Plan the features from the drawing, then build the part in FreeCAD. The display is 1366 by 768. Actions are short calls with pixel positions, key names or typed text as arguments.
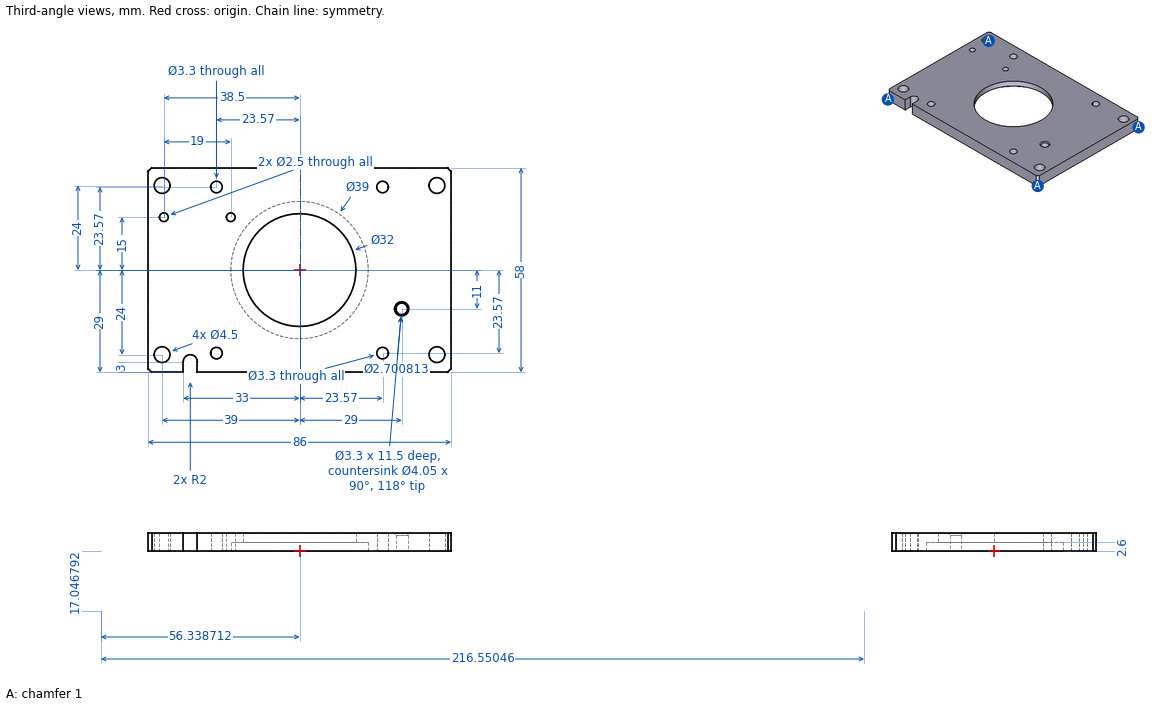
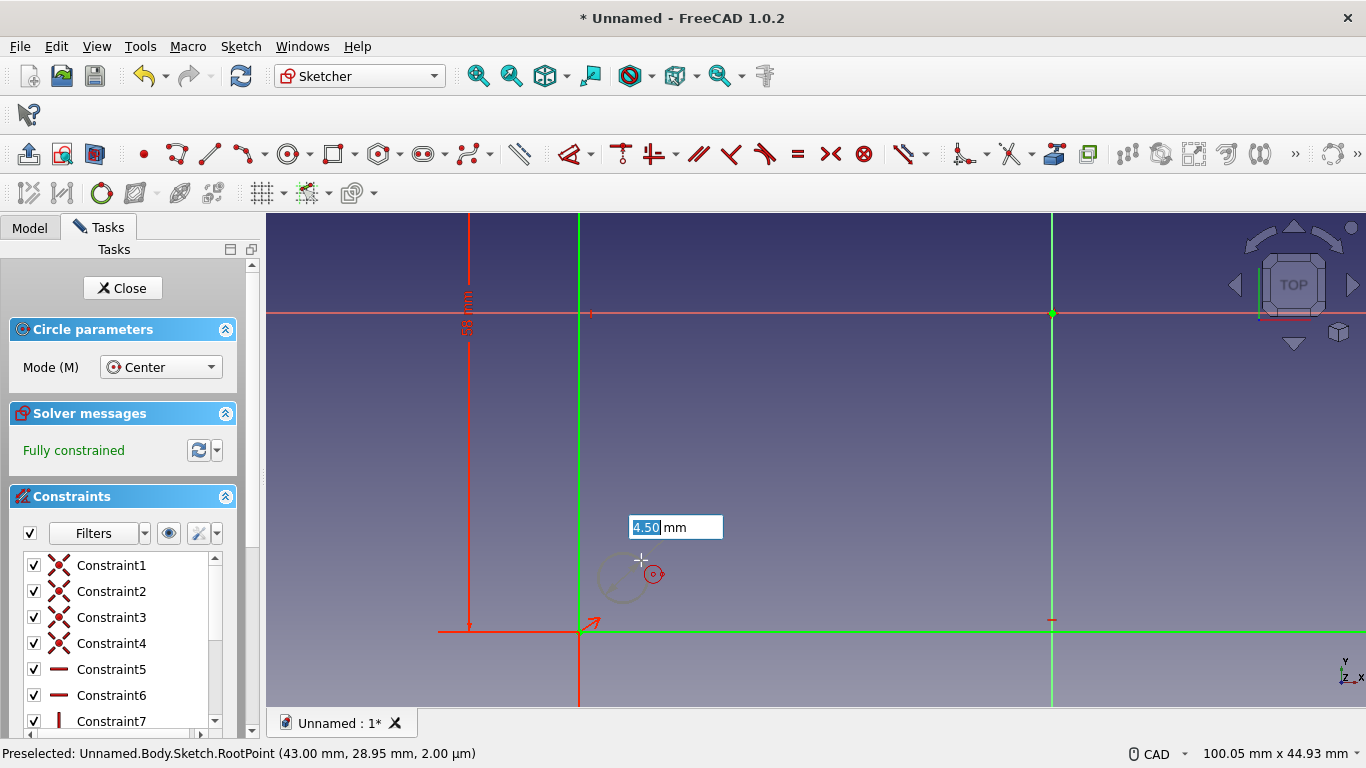
text(4.5)
key(Return)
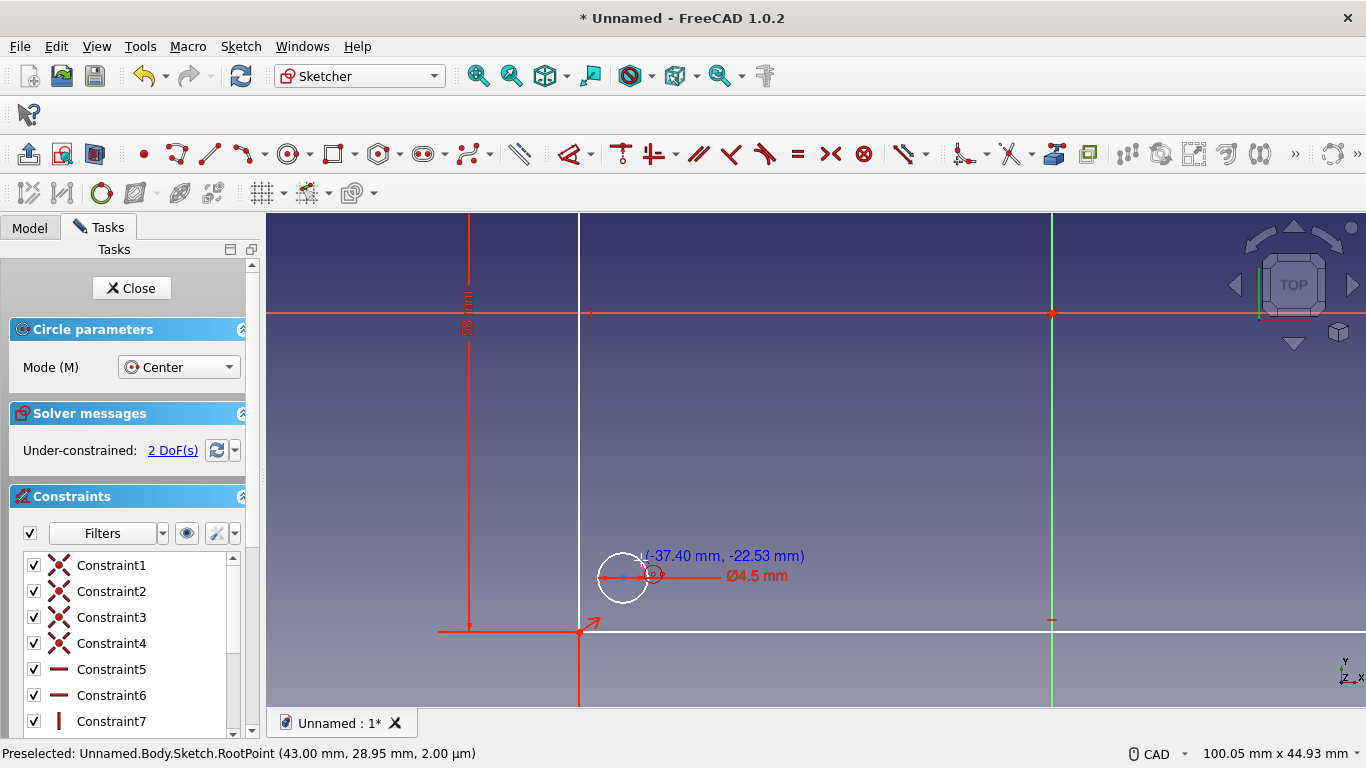
scroll(499, 580, down, 4)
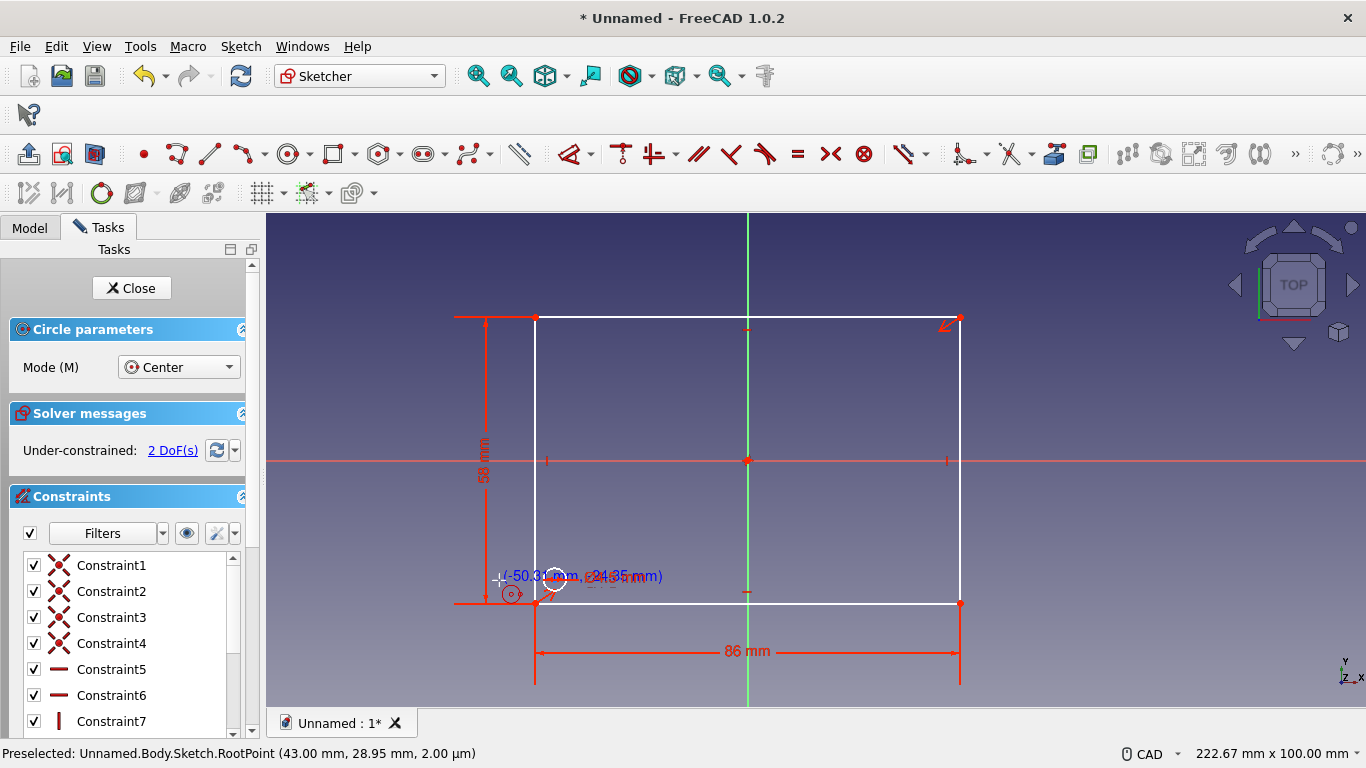
scroll(940, 579, up, 4)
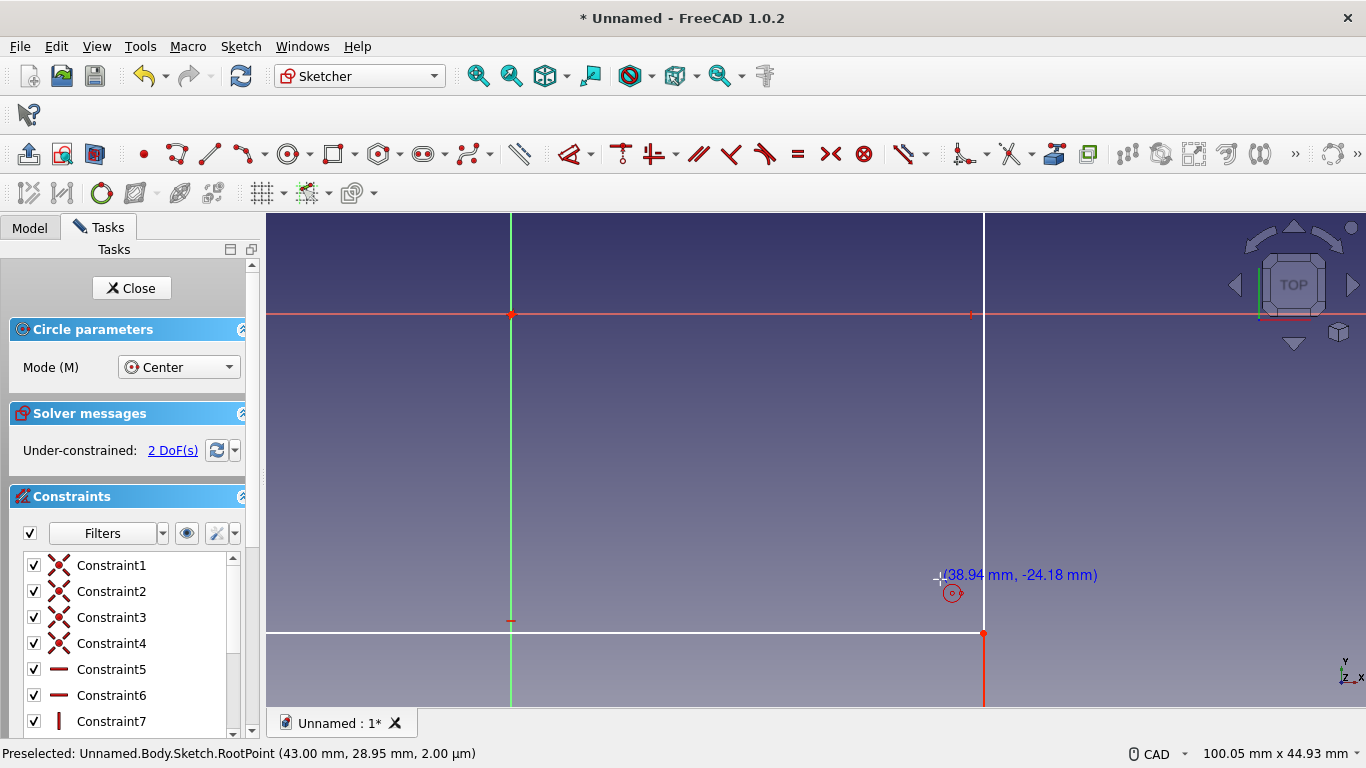
click(940, 578)
move(957, 561)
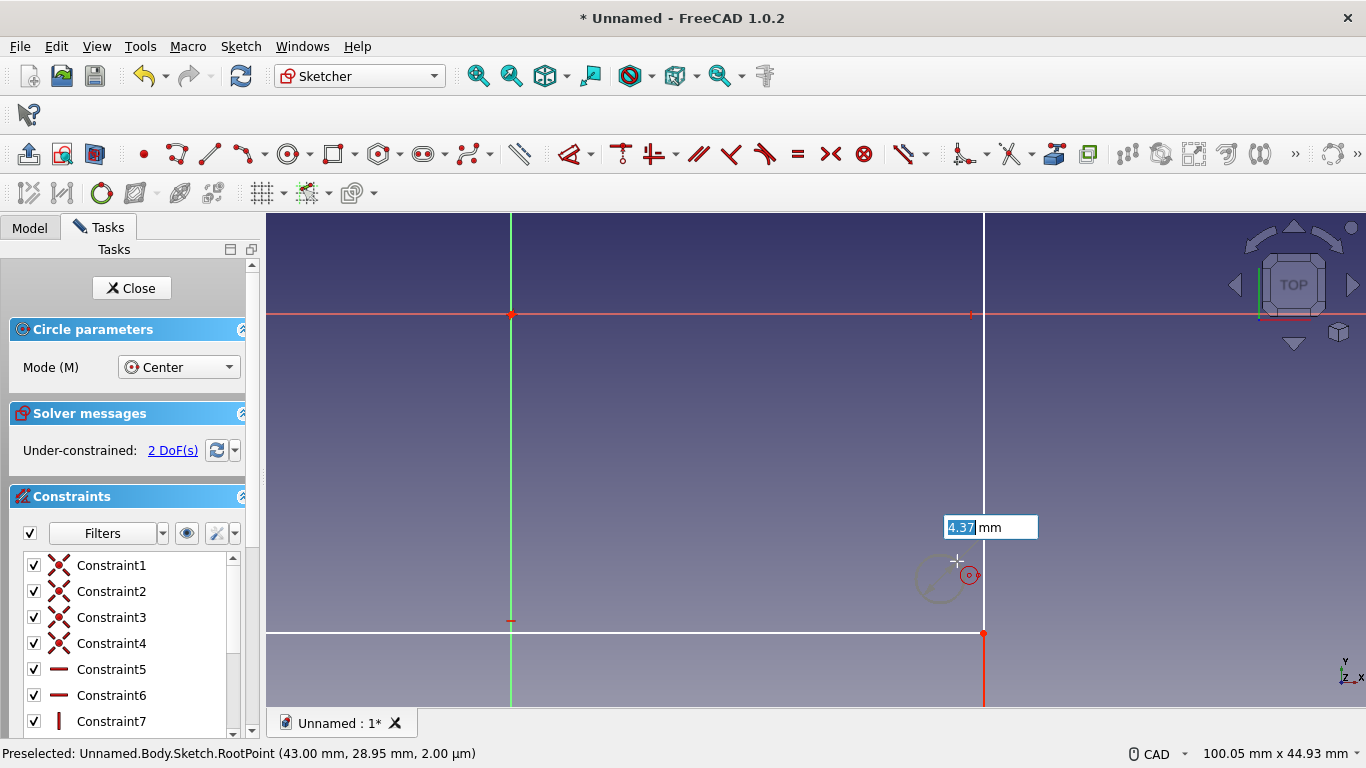
text(4.5)
key(Return)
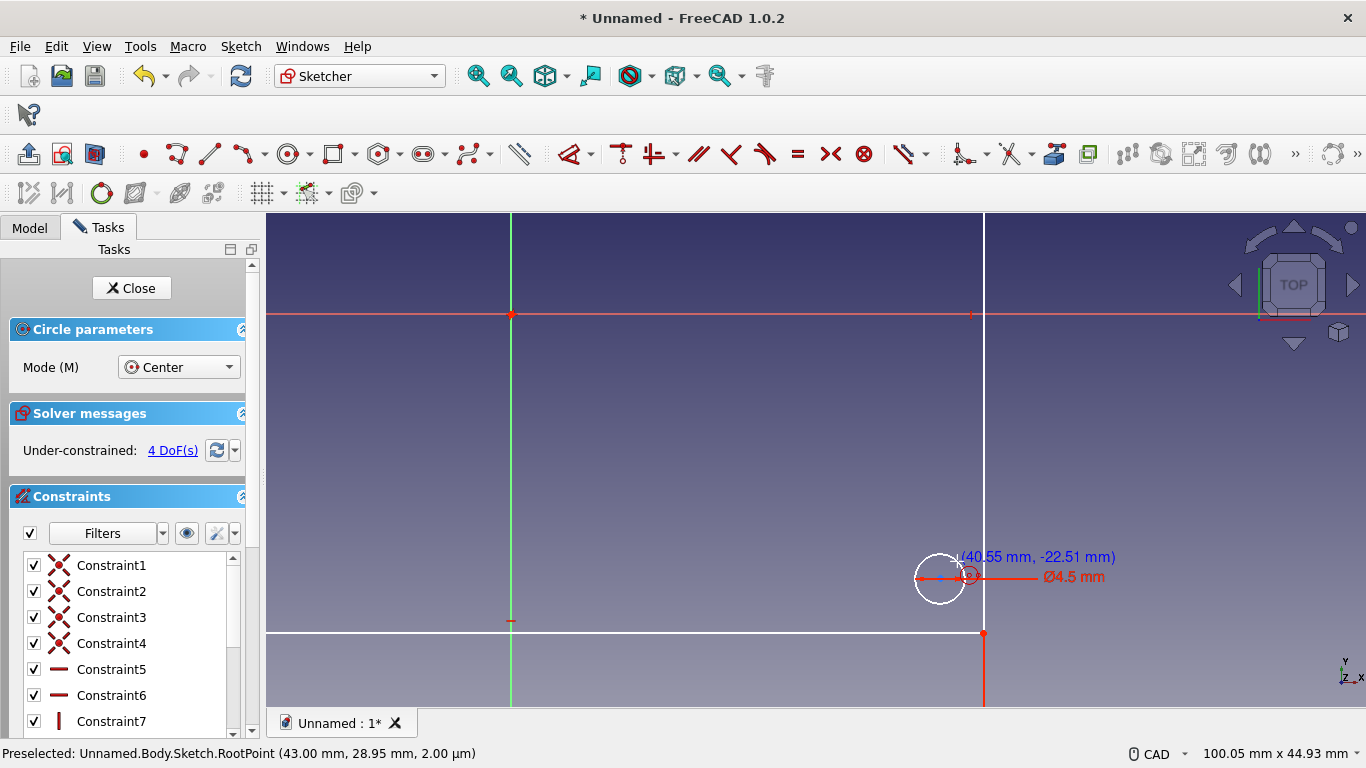
scroll(940, 579, down, 4)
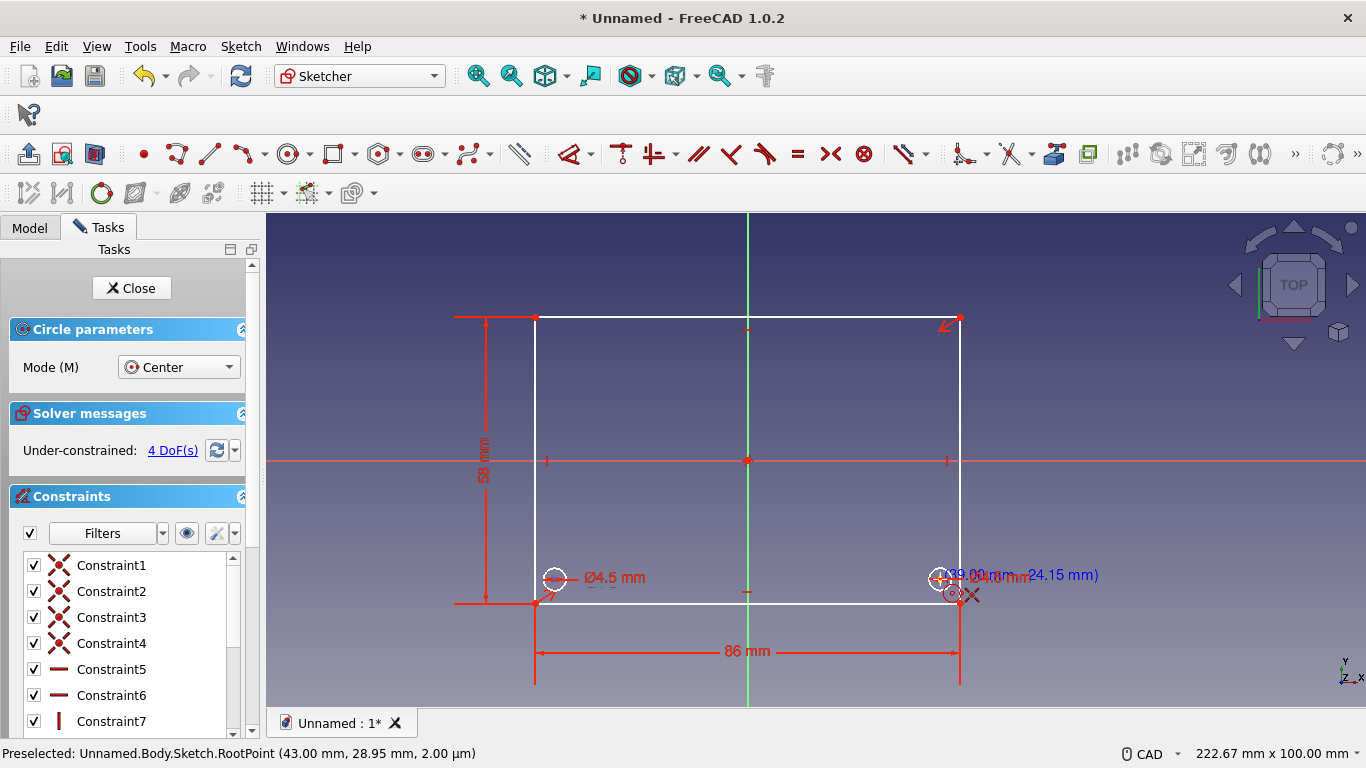
scroll(555, 342, up, 4)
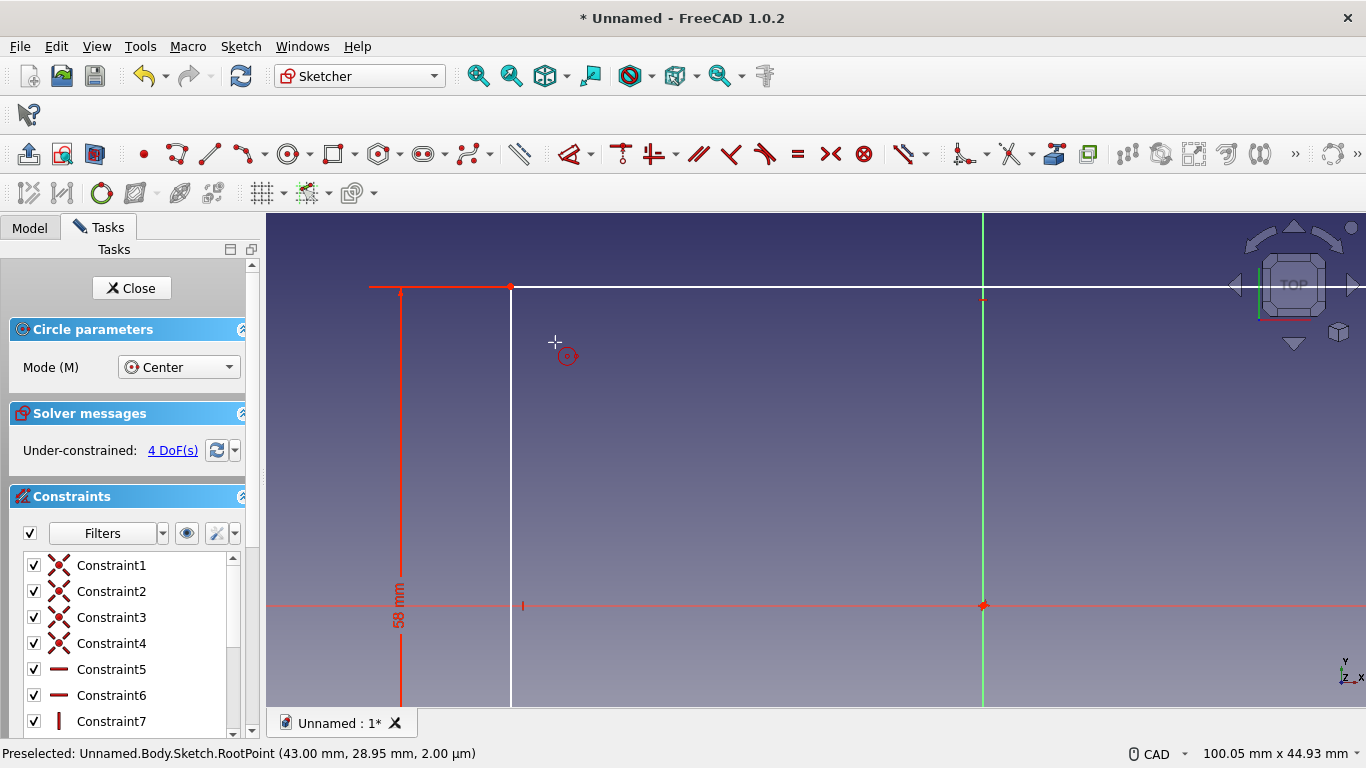
click(555, 342)
move(572, 324)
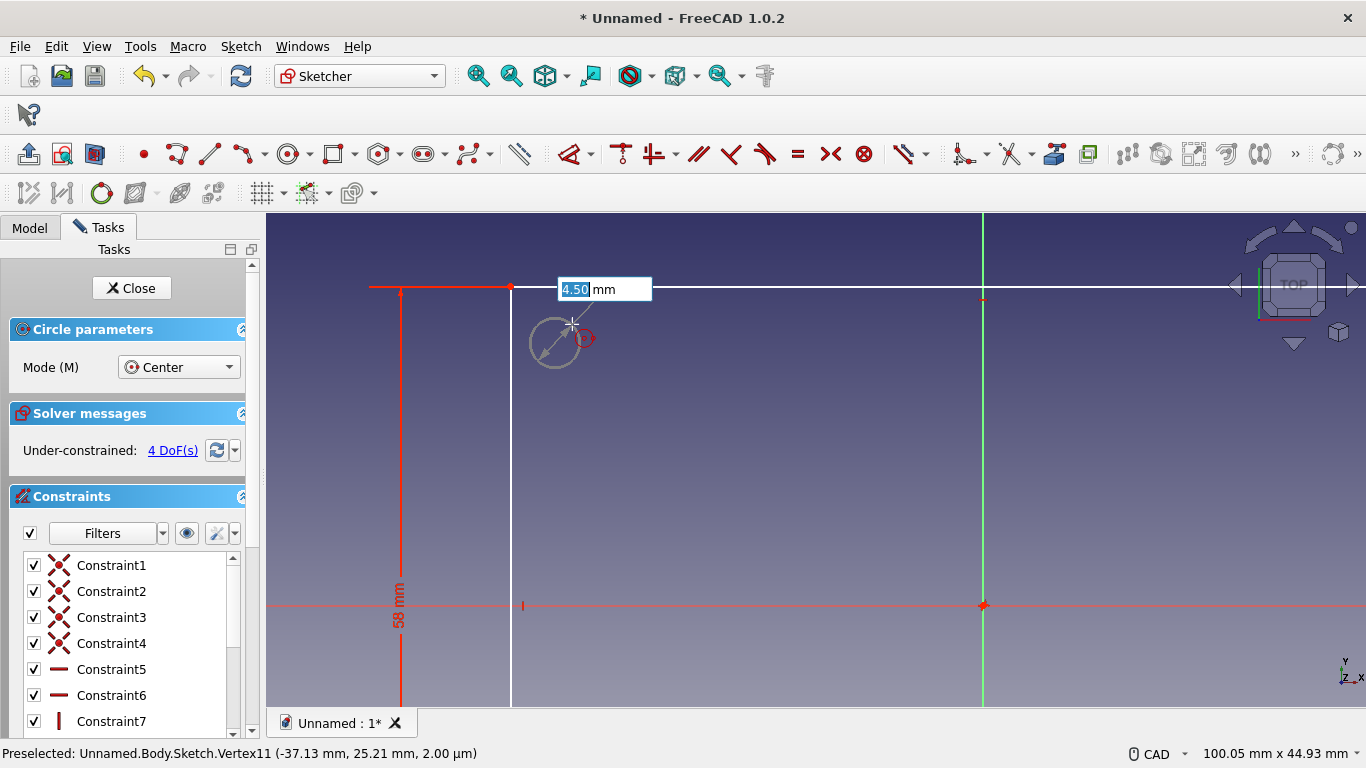
text(4.5)
key(Return)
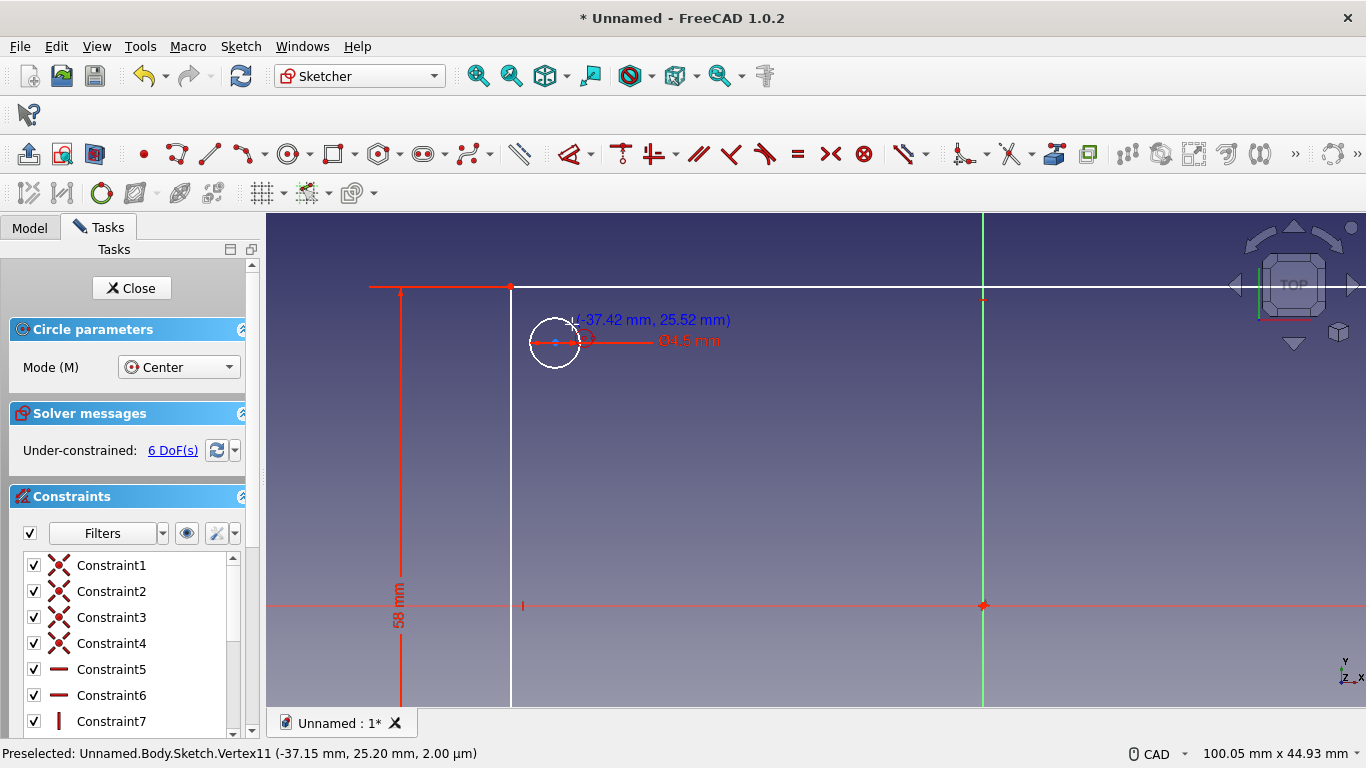
click(983, 606)
move(1108, 481)